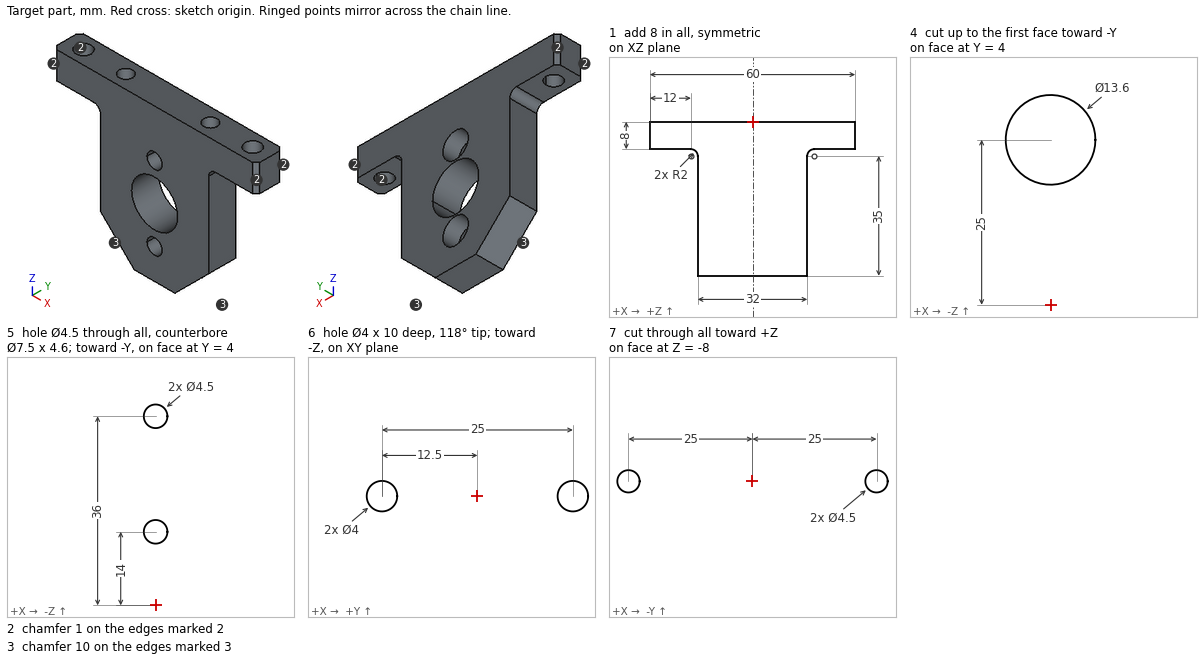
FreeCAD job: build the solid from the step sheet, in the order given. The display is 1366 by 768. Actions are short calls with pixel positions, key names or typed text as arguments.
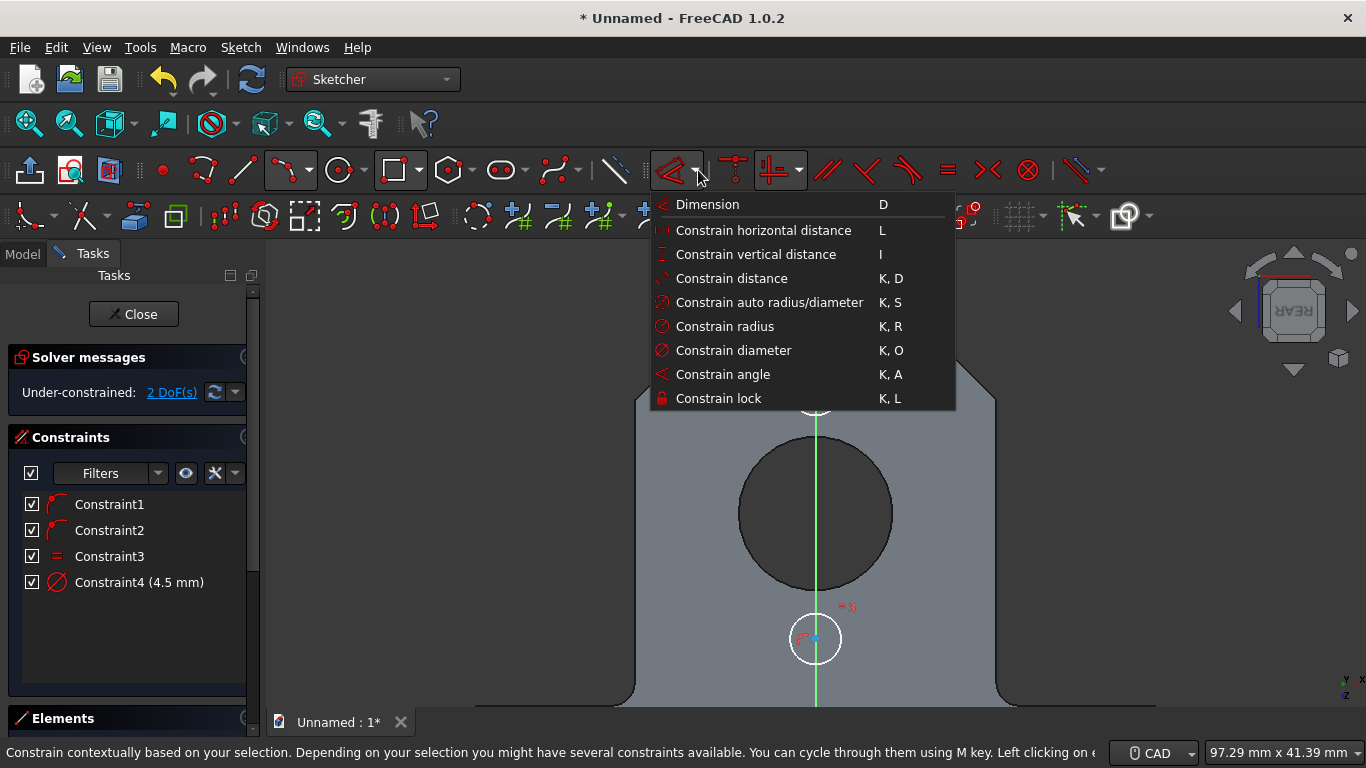
click(803, 254)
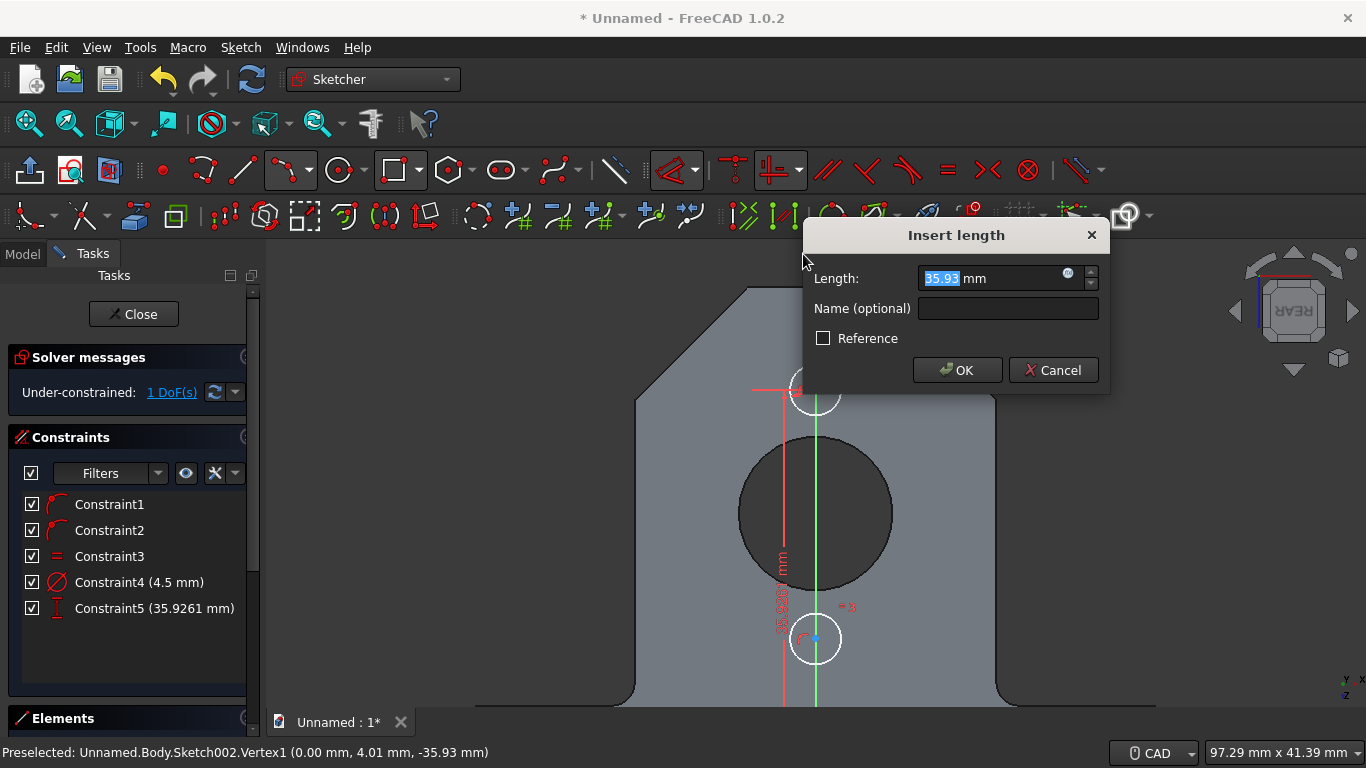
text(36)
key(Return)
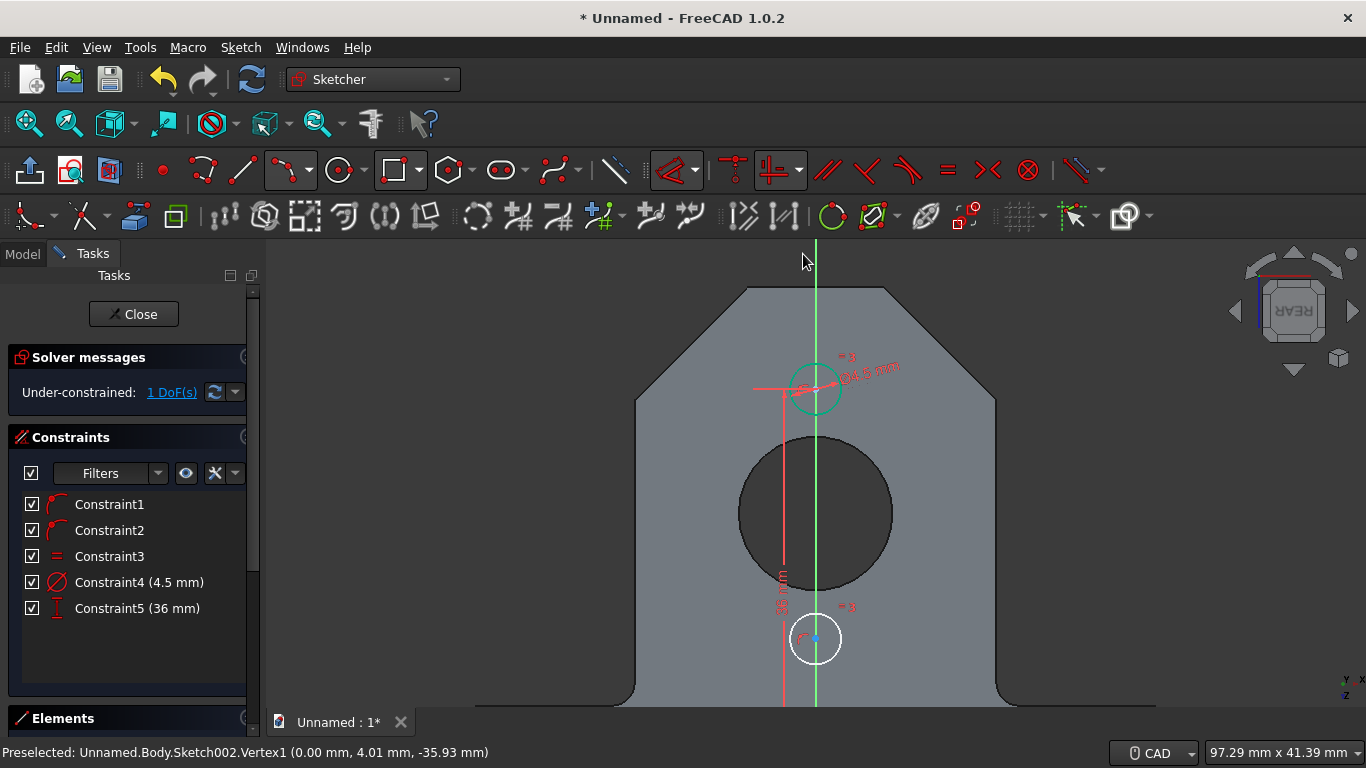
click(816, 639)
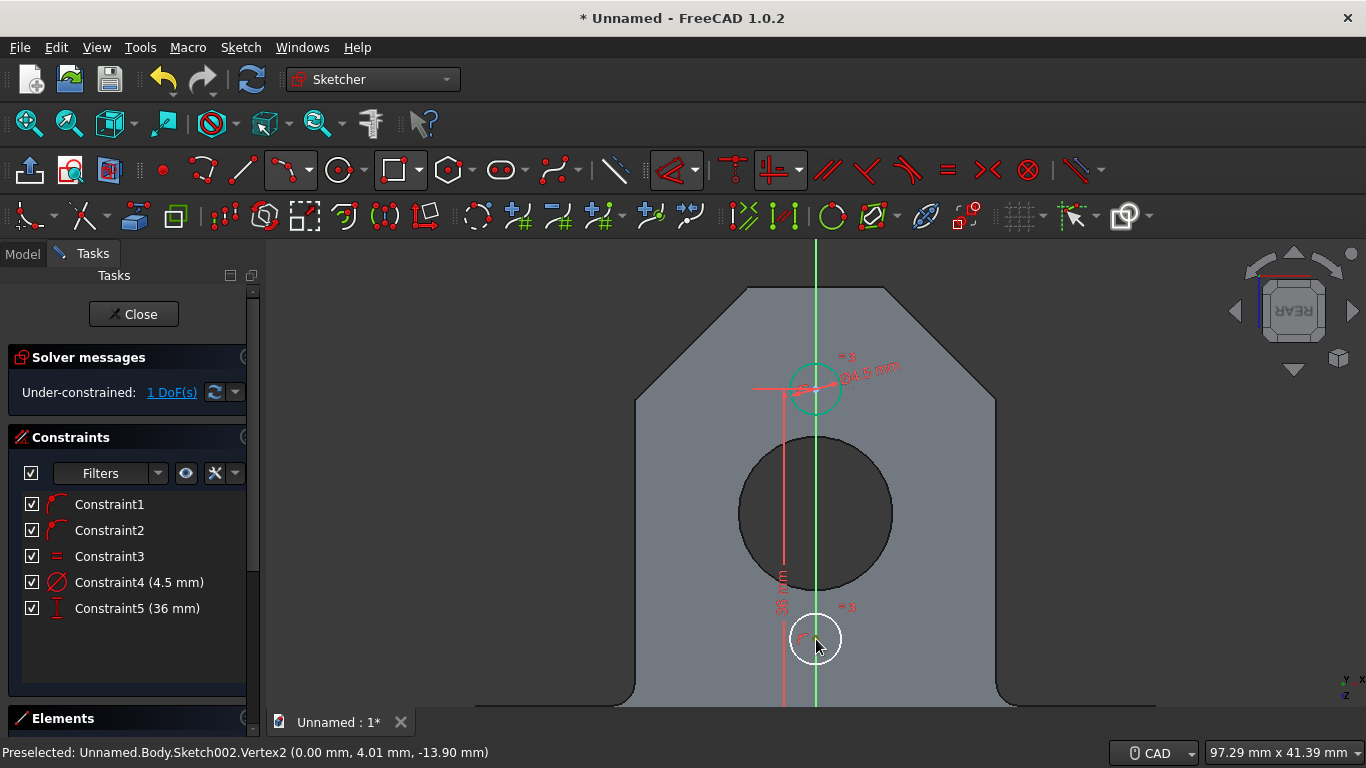
key(i)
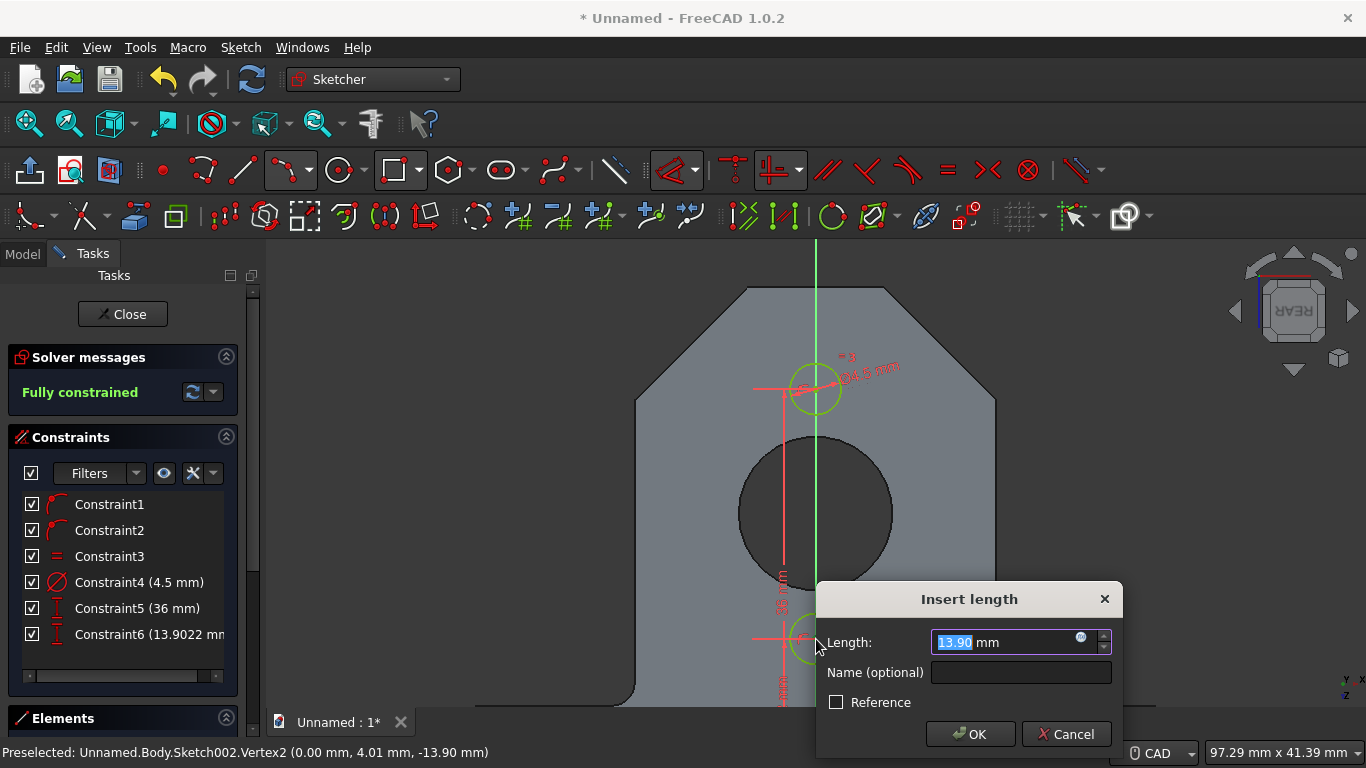
text(14)
key(Return)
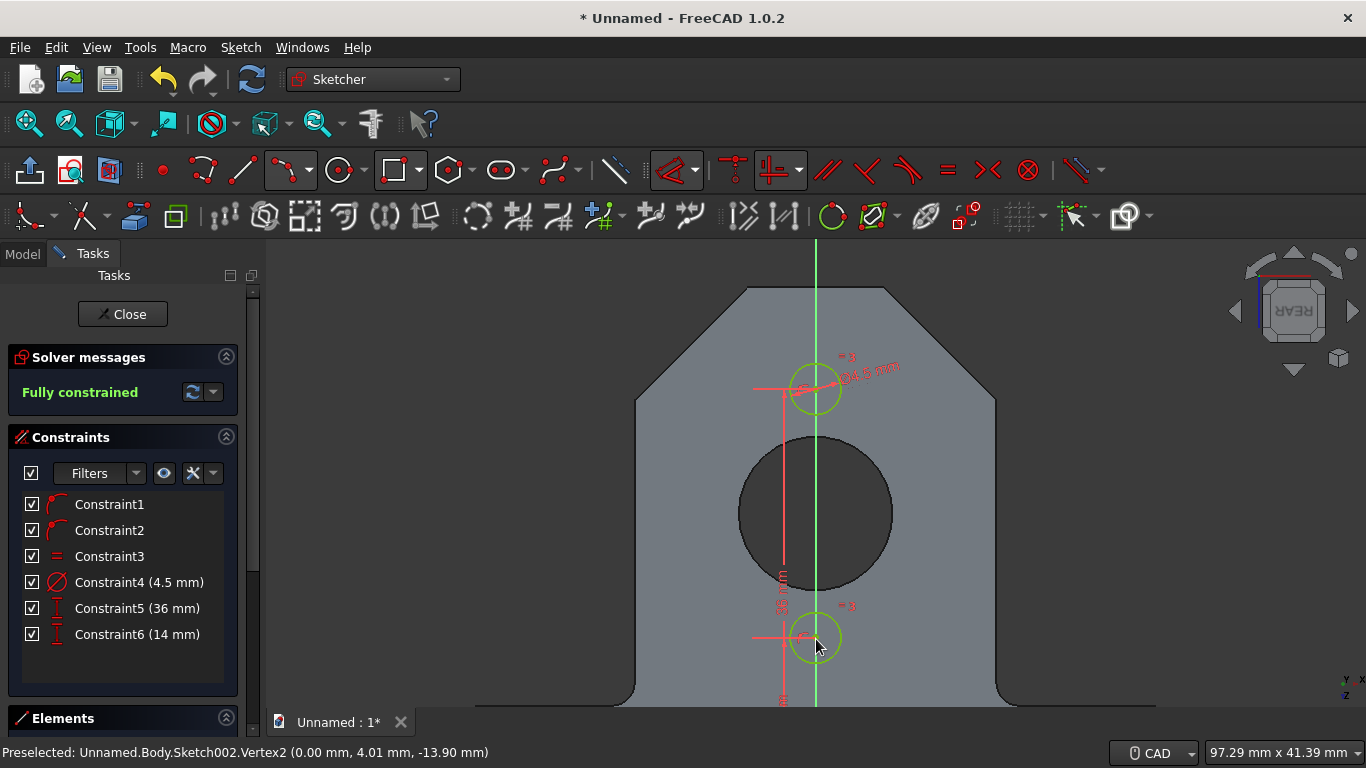
click(123, 314)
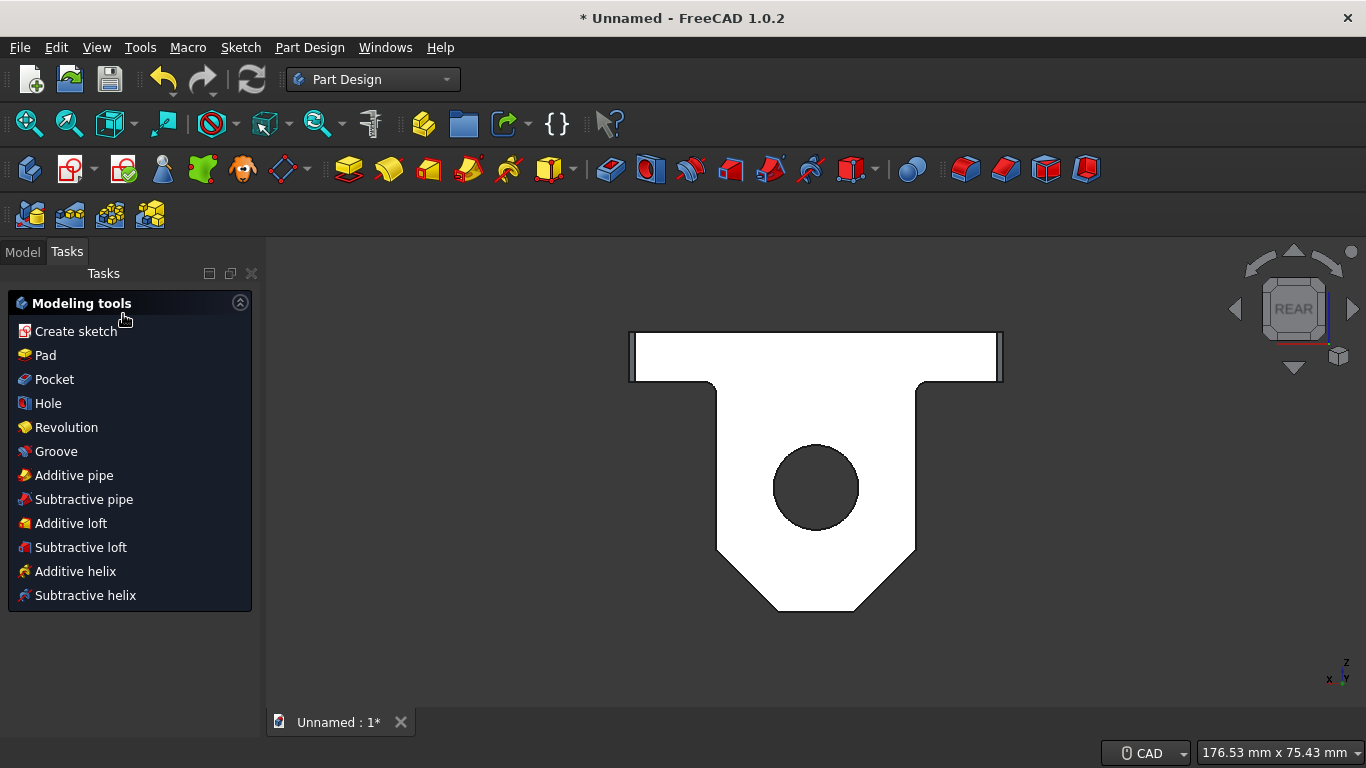
click(652, 170)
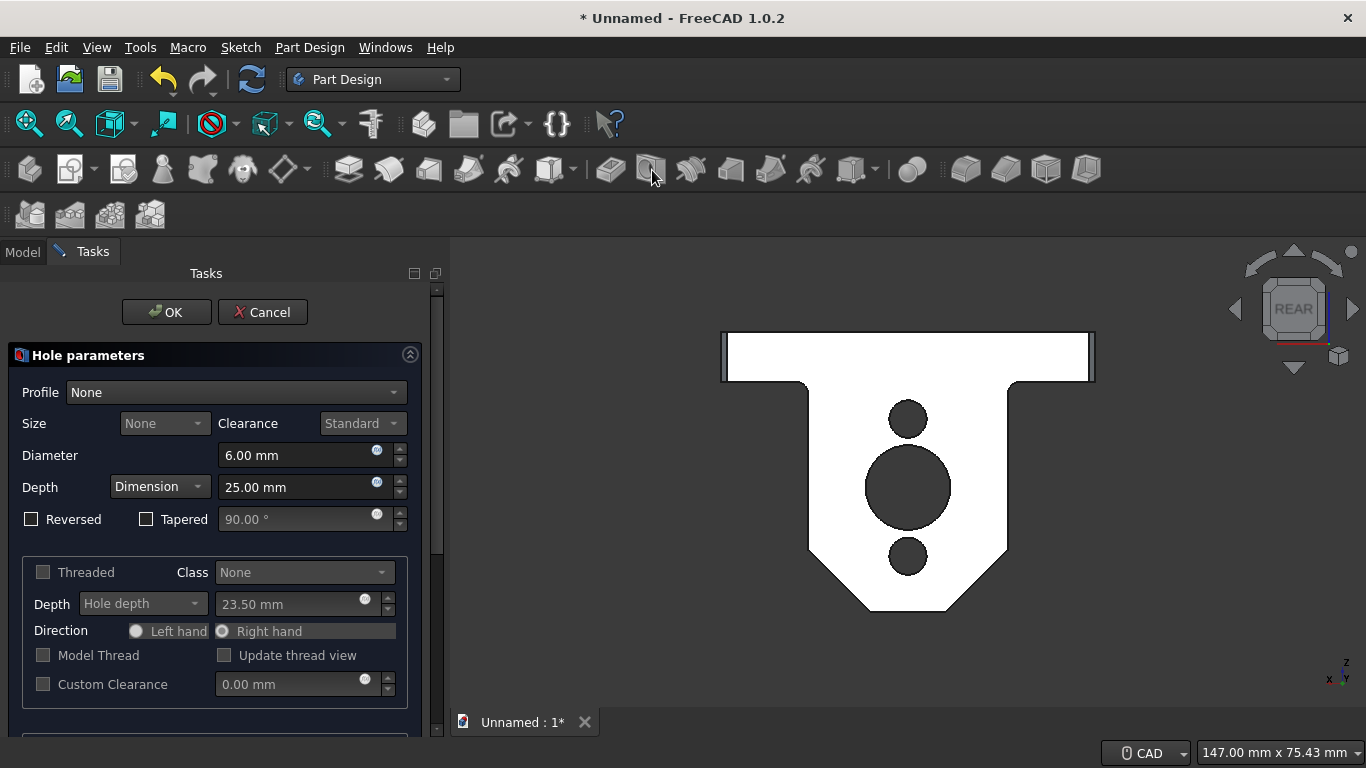
triple_click(305, 455)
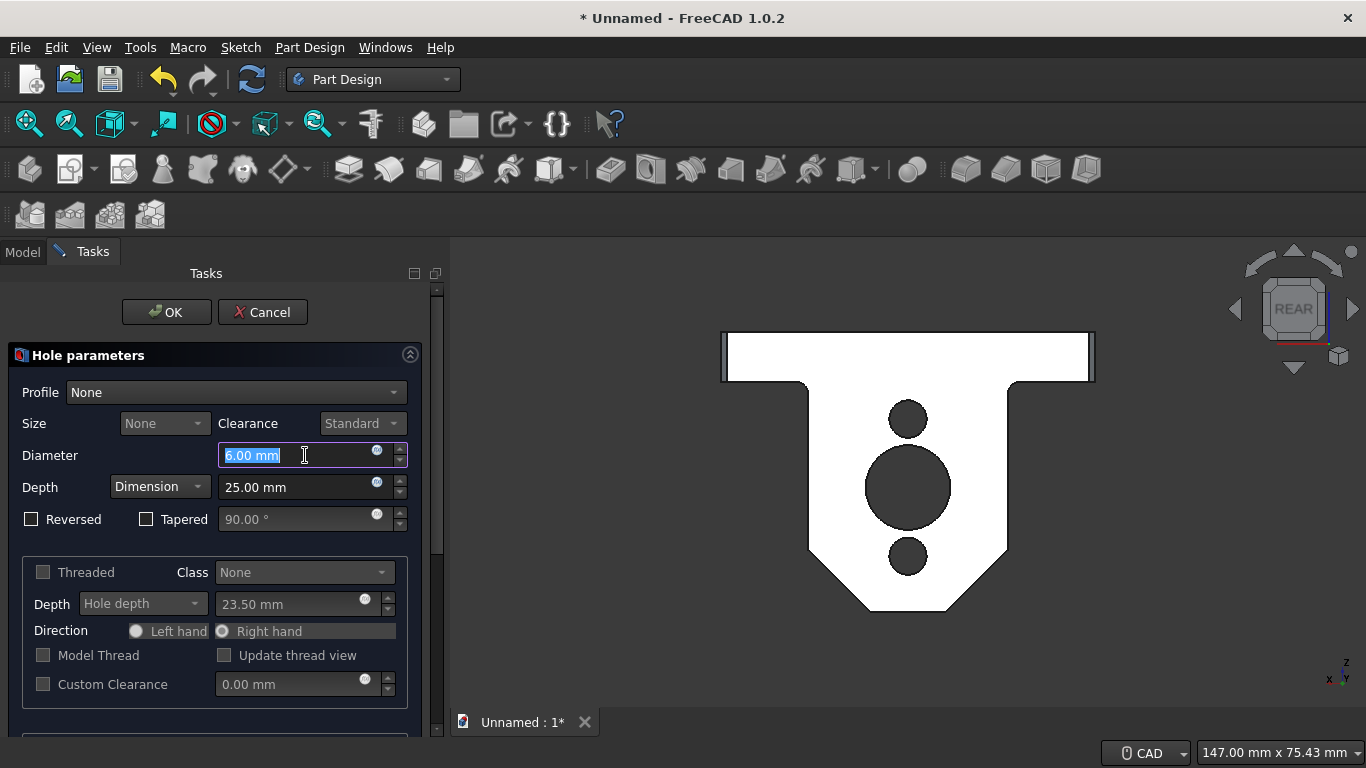
text(4.5)
key(Tab)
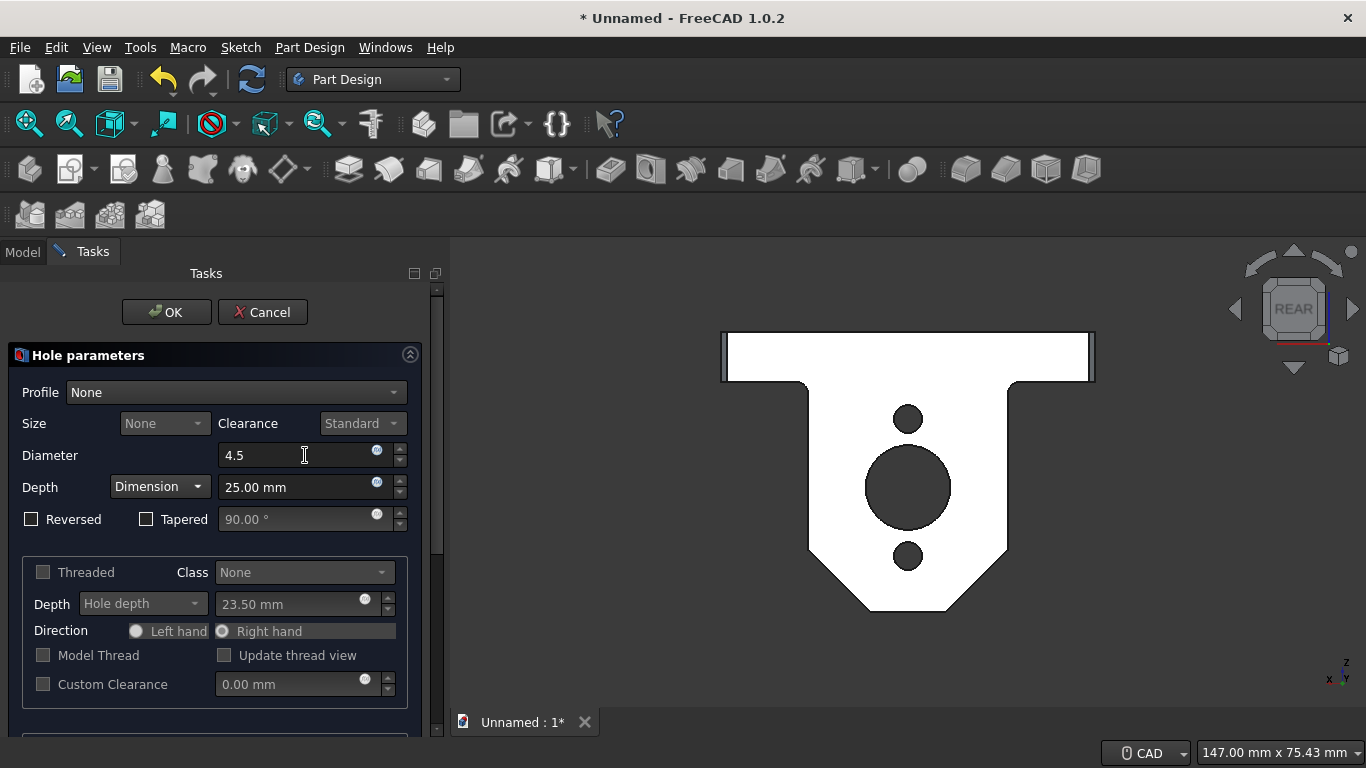
click(161, 486)